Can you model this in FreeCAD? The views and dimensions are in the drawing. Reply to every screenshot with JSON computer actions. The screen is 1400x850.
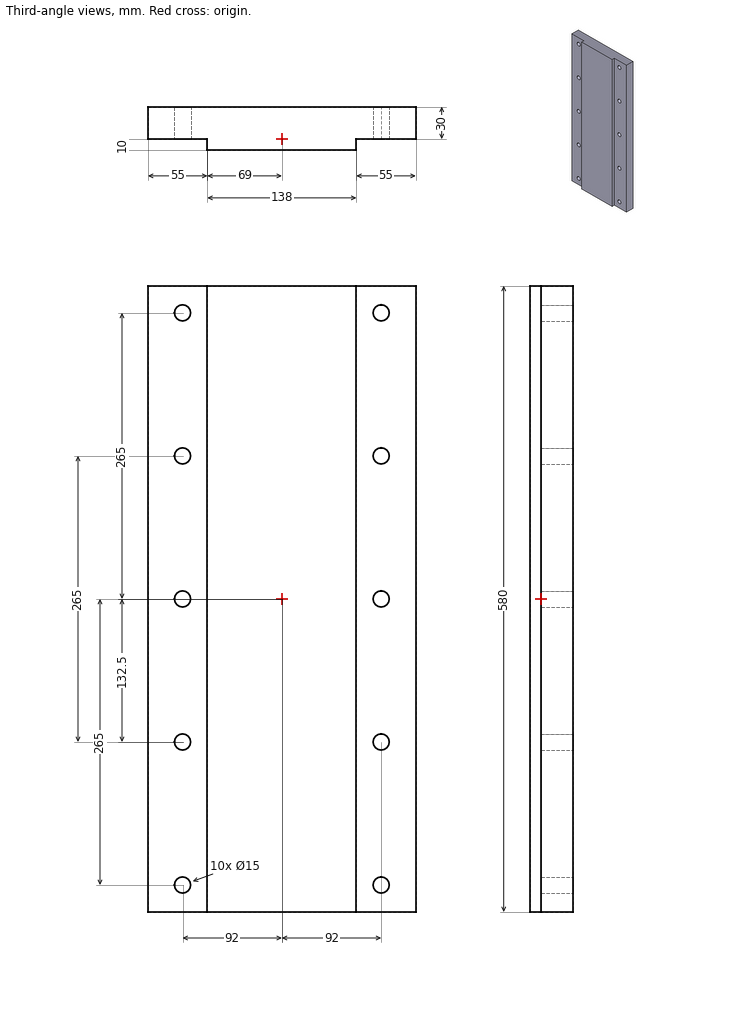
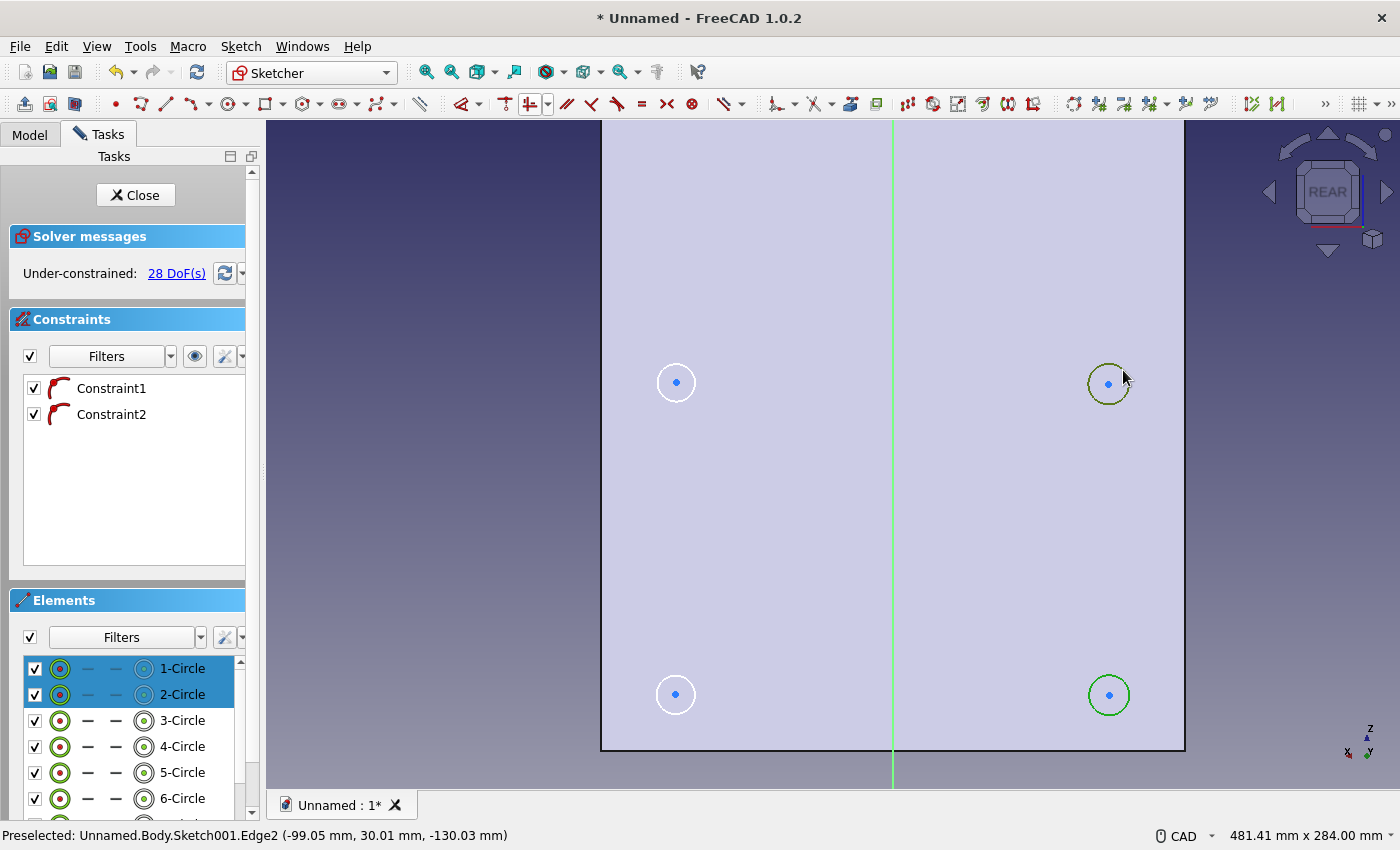
{"action": "scroll", "coordinate": [690, 679], "scroll_direction": "down", "scroll_amount": 5}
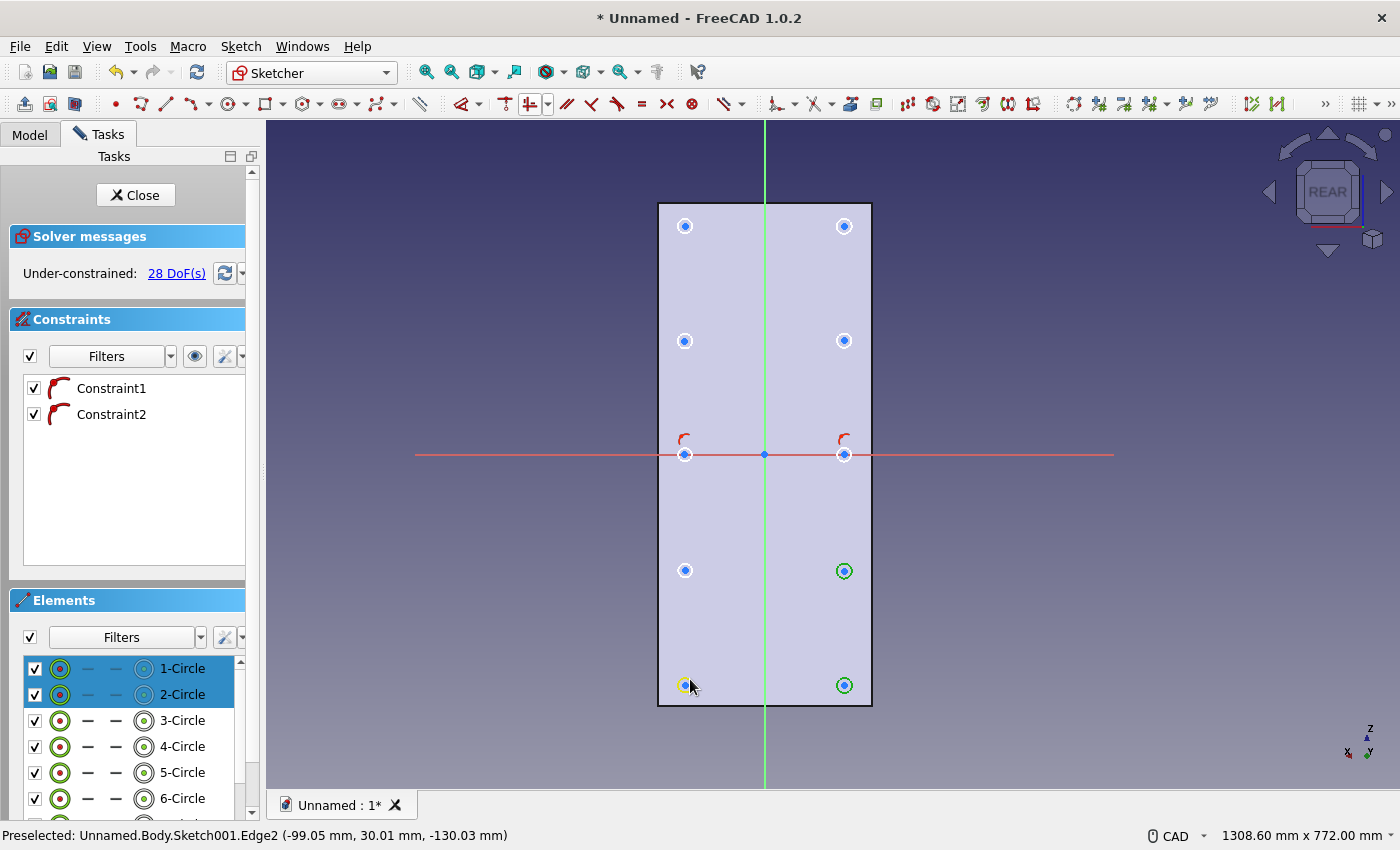
{"action": "scroll", "coordinate": [849, 450], "scroll_direction": "up", "scroll_amount": 6}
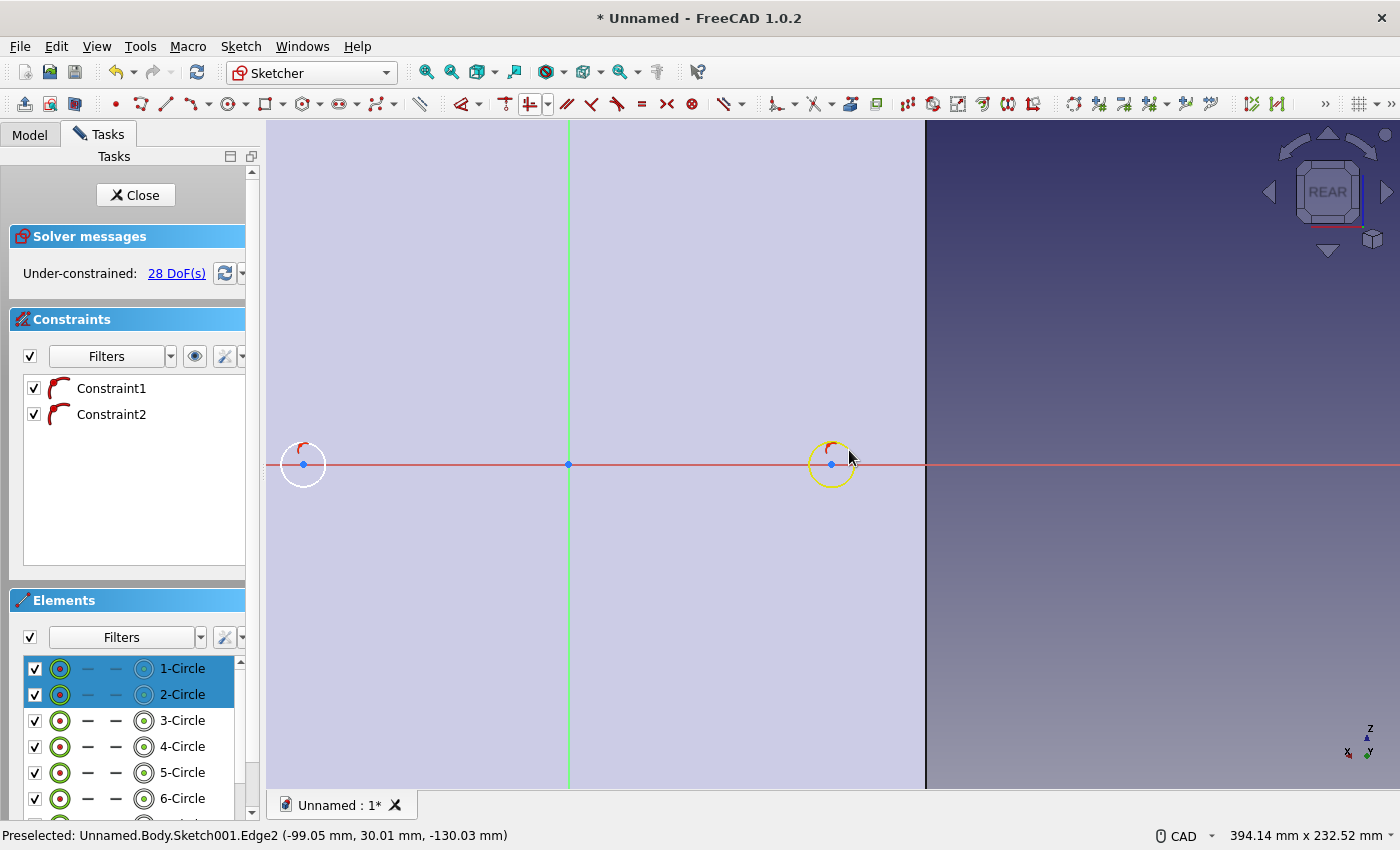
{"action": "left_click", "coordinate": [848, 449]}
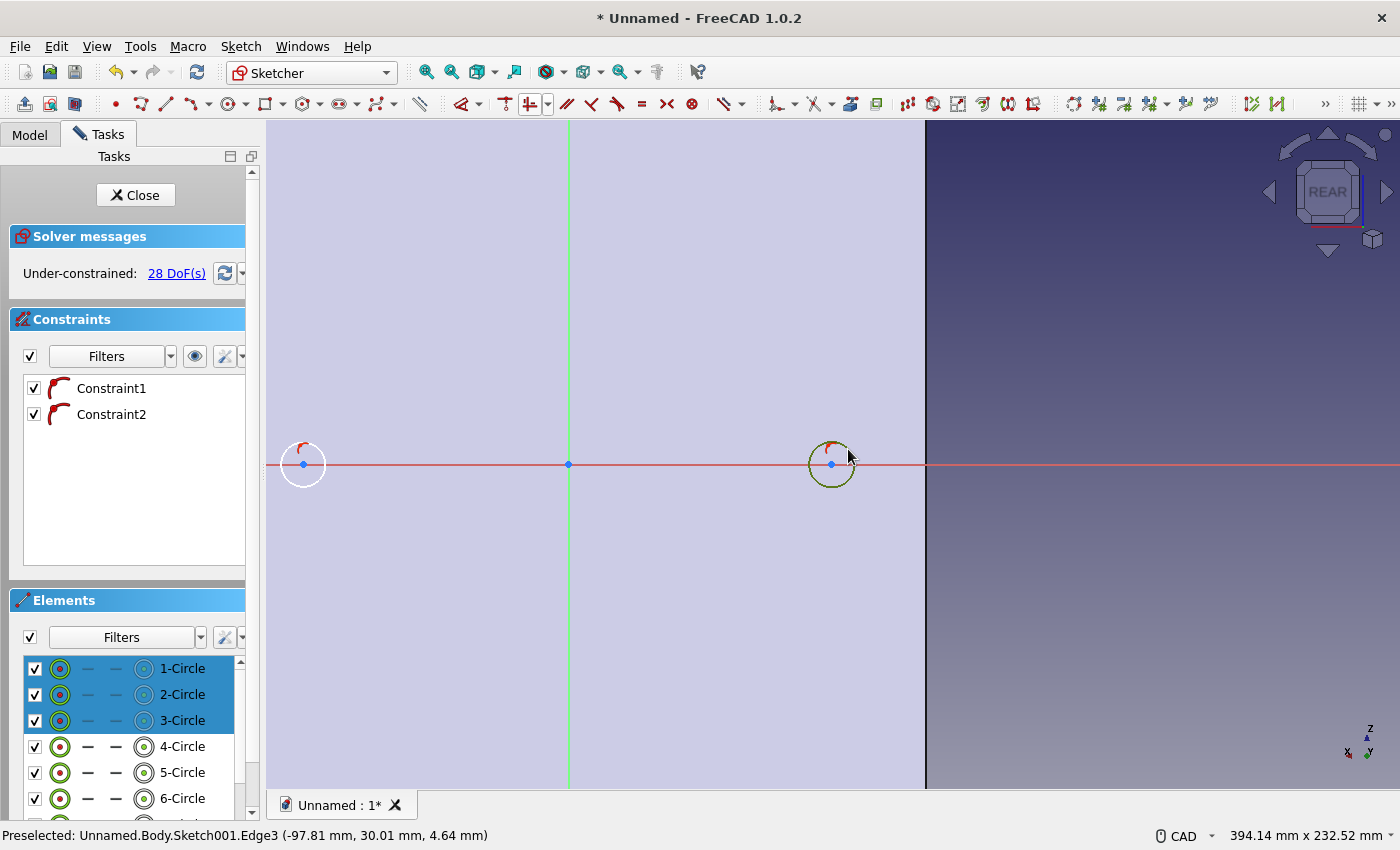
{"action": "scroll", "coordinate": [849, 450], "scroll_direction": "down", "scroll_amount": 6}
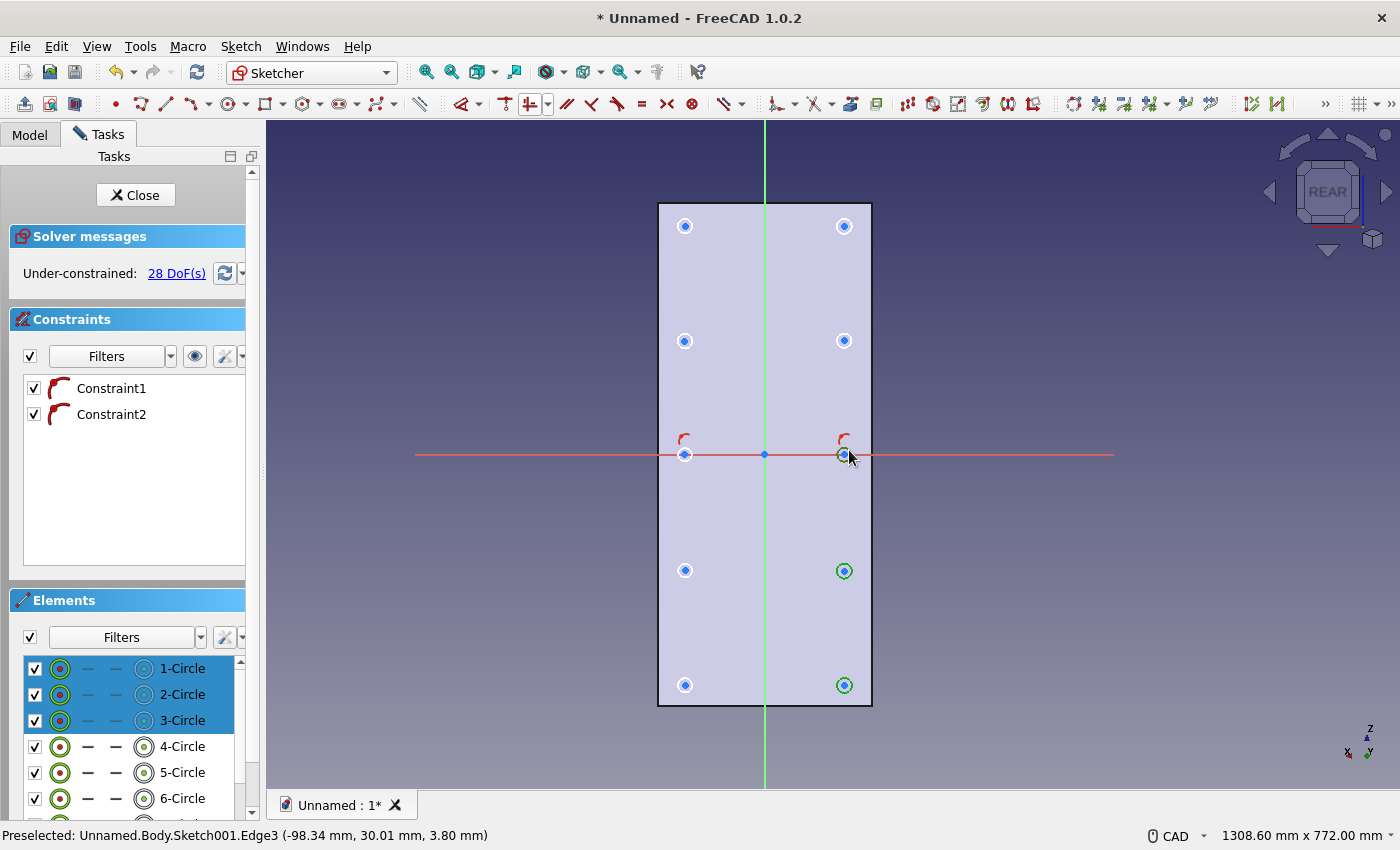
{"action": "scroll", "coordinate": [849, 336], "scroll_direction": "up", "scroll_amount": 4}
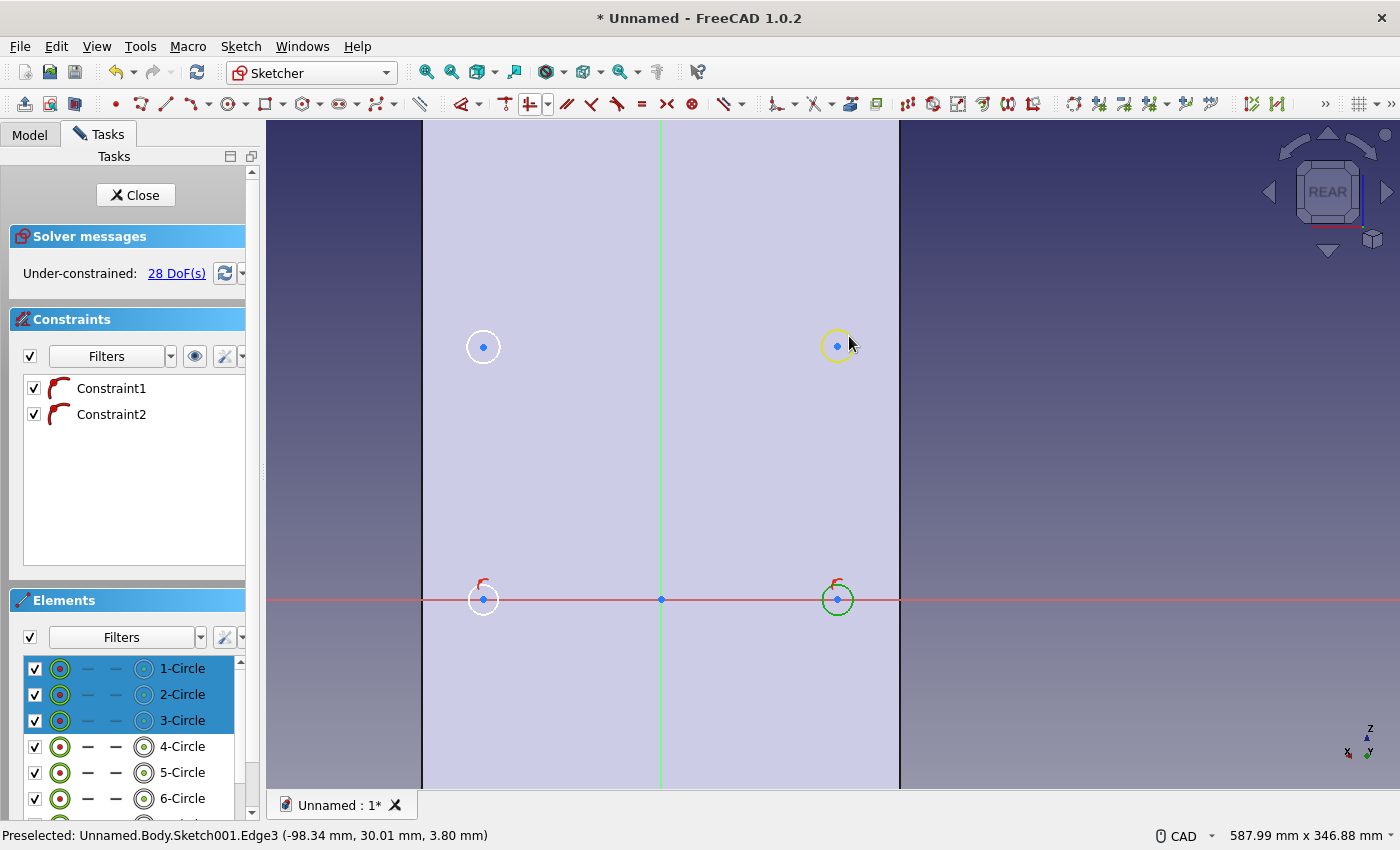
{"action": "left_click", "coordinate": [849, 335]}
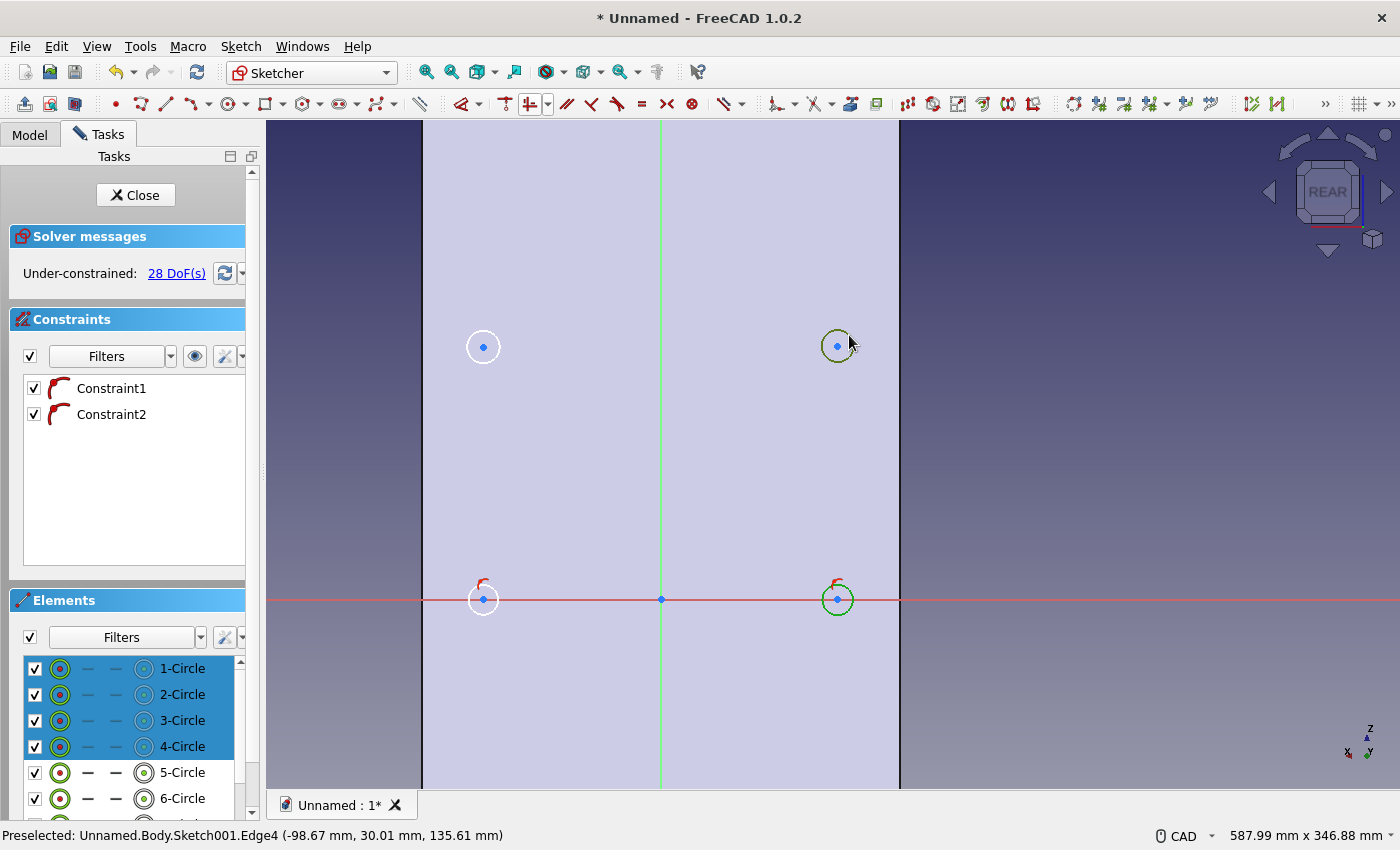
{"action": "scroll", "coordinate": [849, 336], "scroll_direction": "down", "scroll_amount": 4}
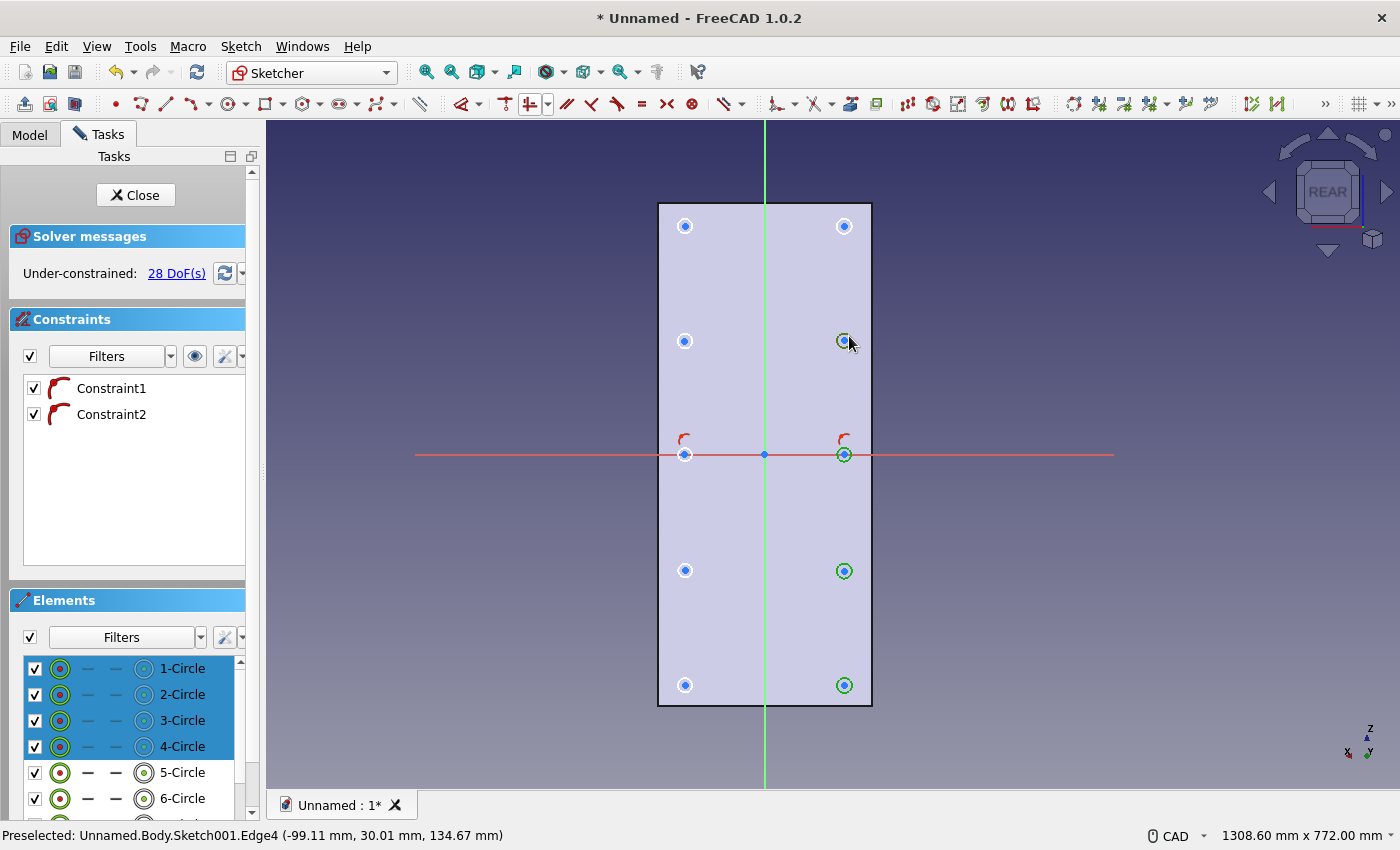
{"action": "scroll", "coordinate": [849, 221], "scroll_direction": "up", "scroll_amount": 4}